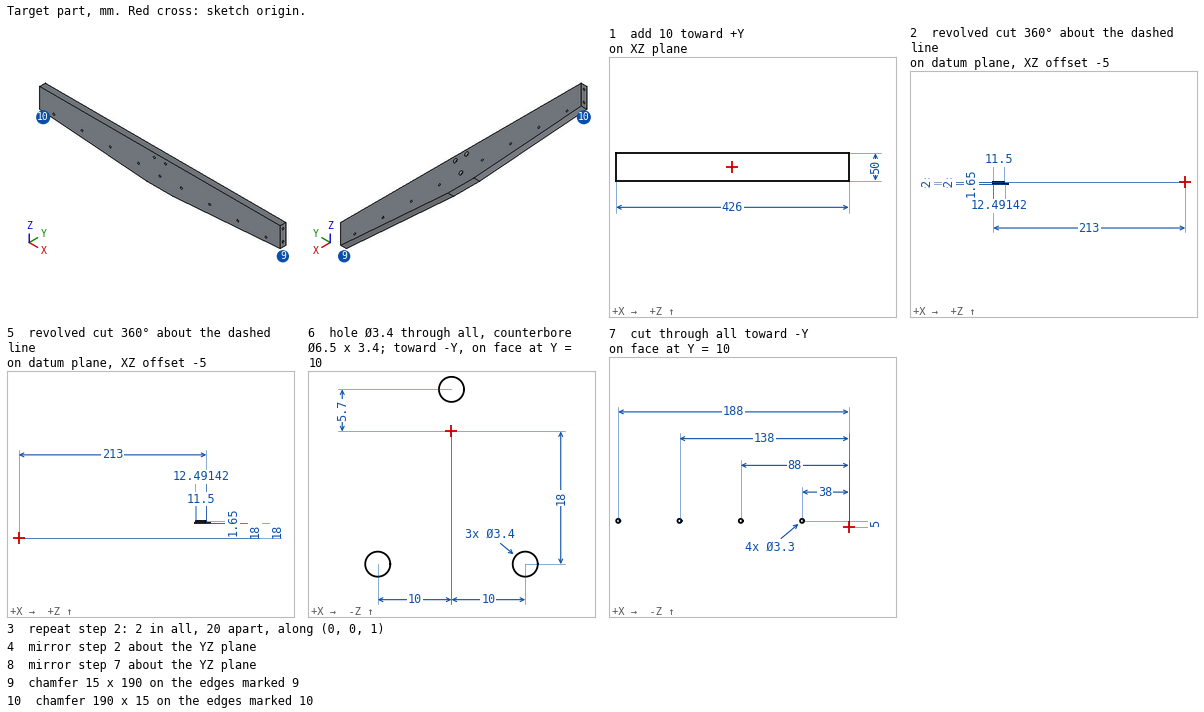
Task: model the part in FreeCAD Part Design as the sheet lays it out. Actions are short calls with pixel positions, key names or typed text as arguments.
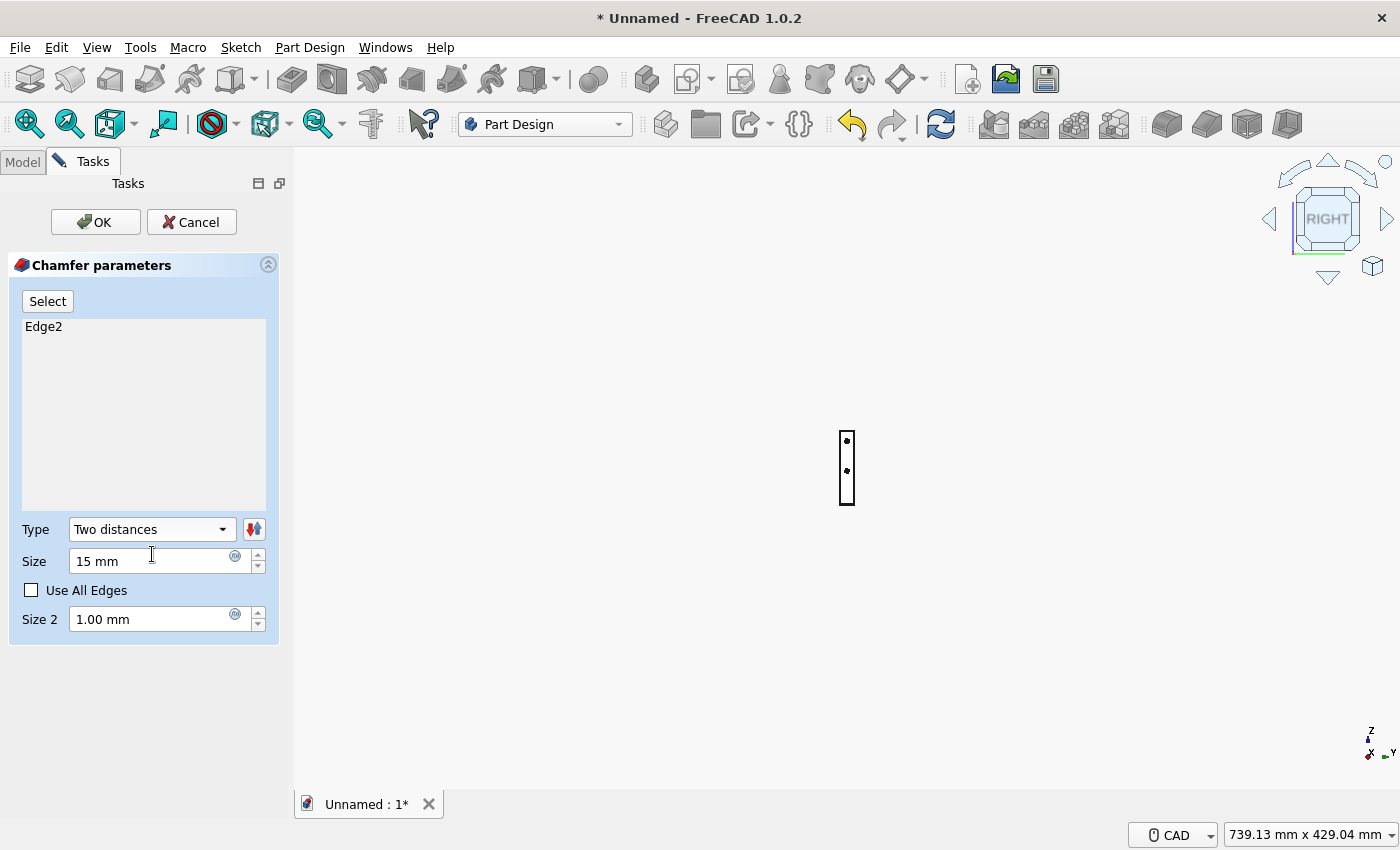
triple_click(160, 619)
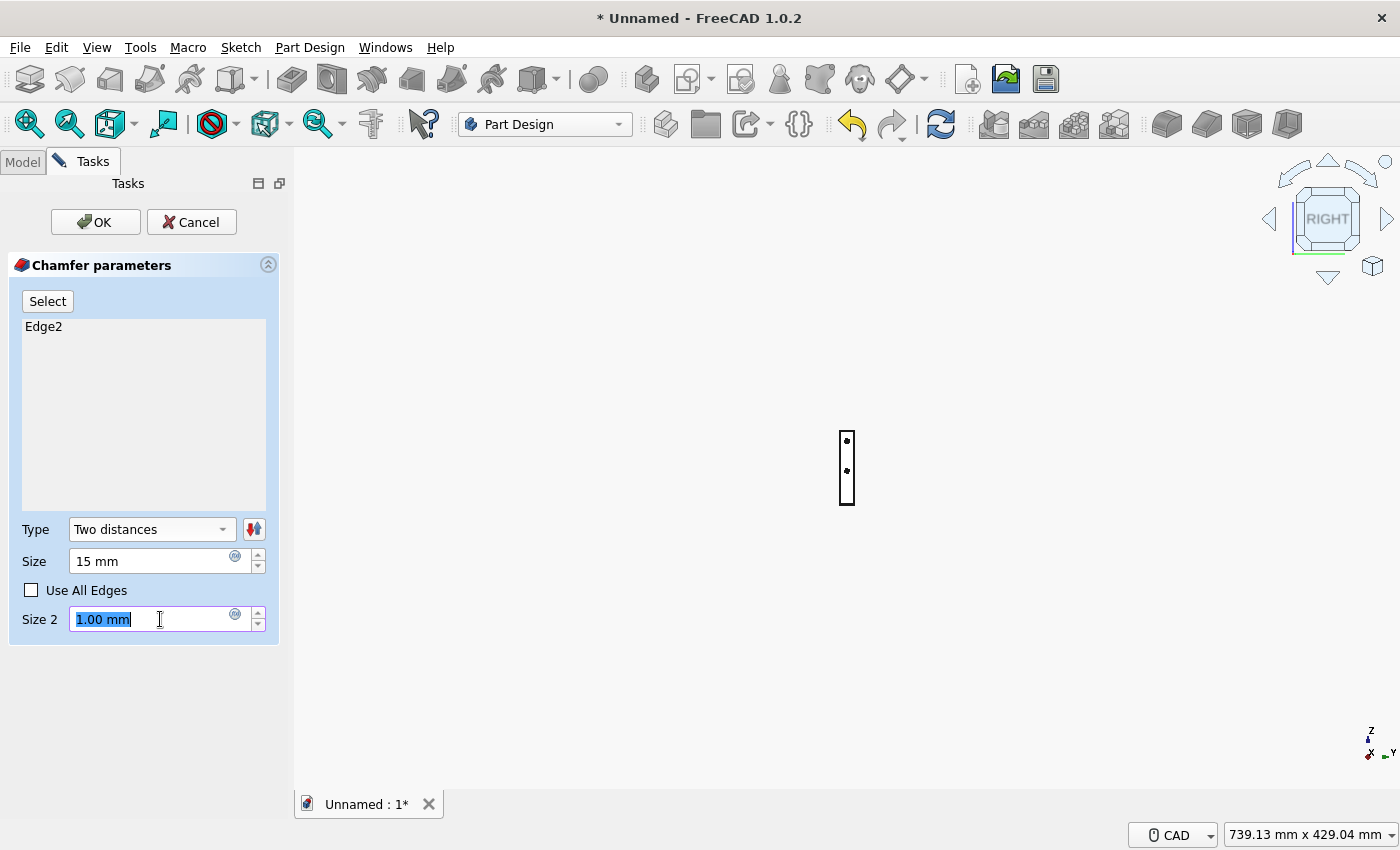
text(190)
key(Tab)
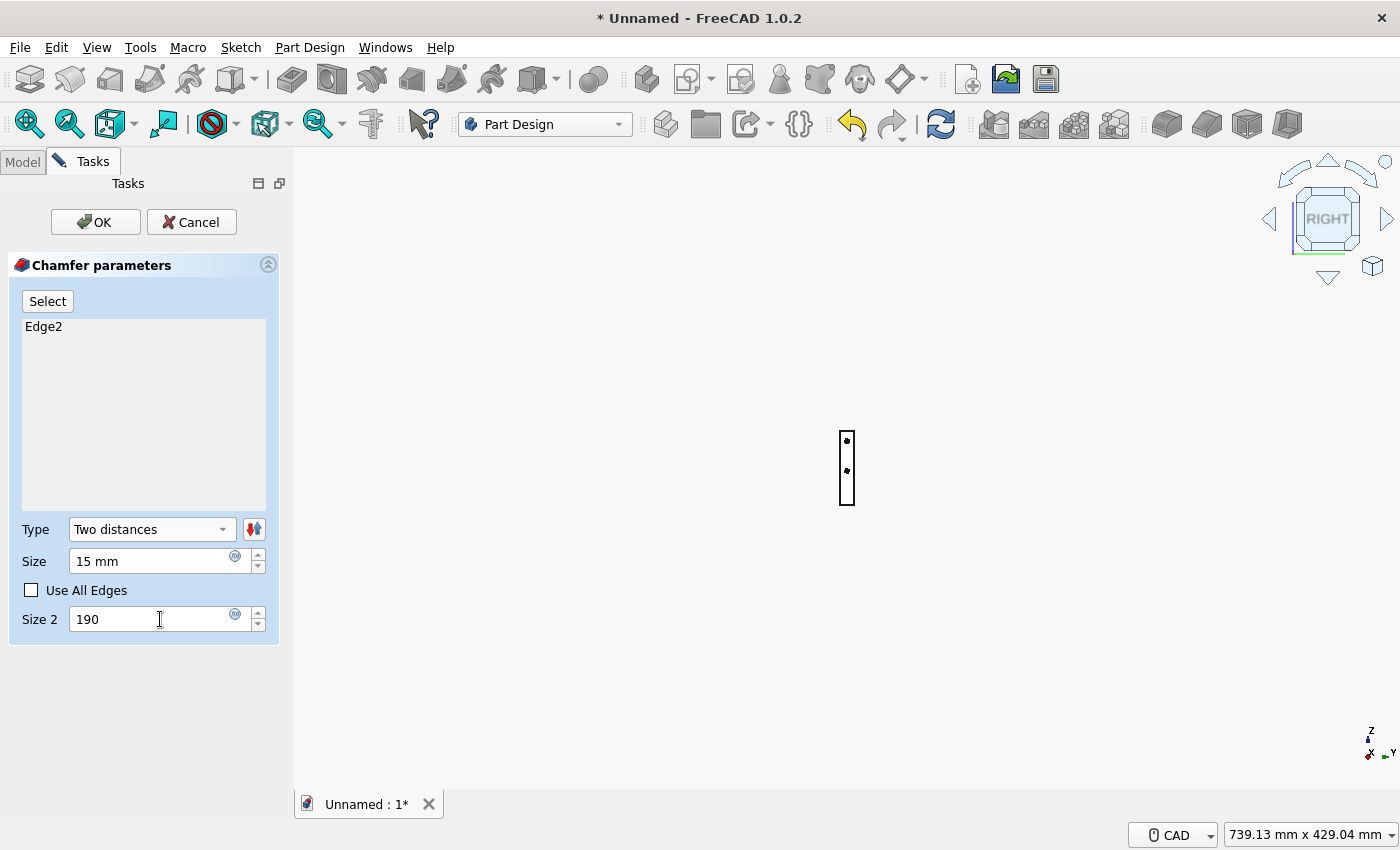
click(254, 530)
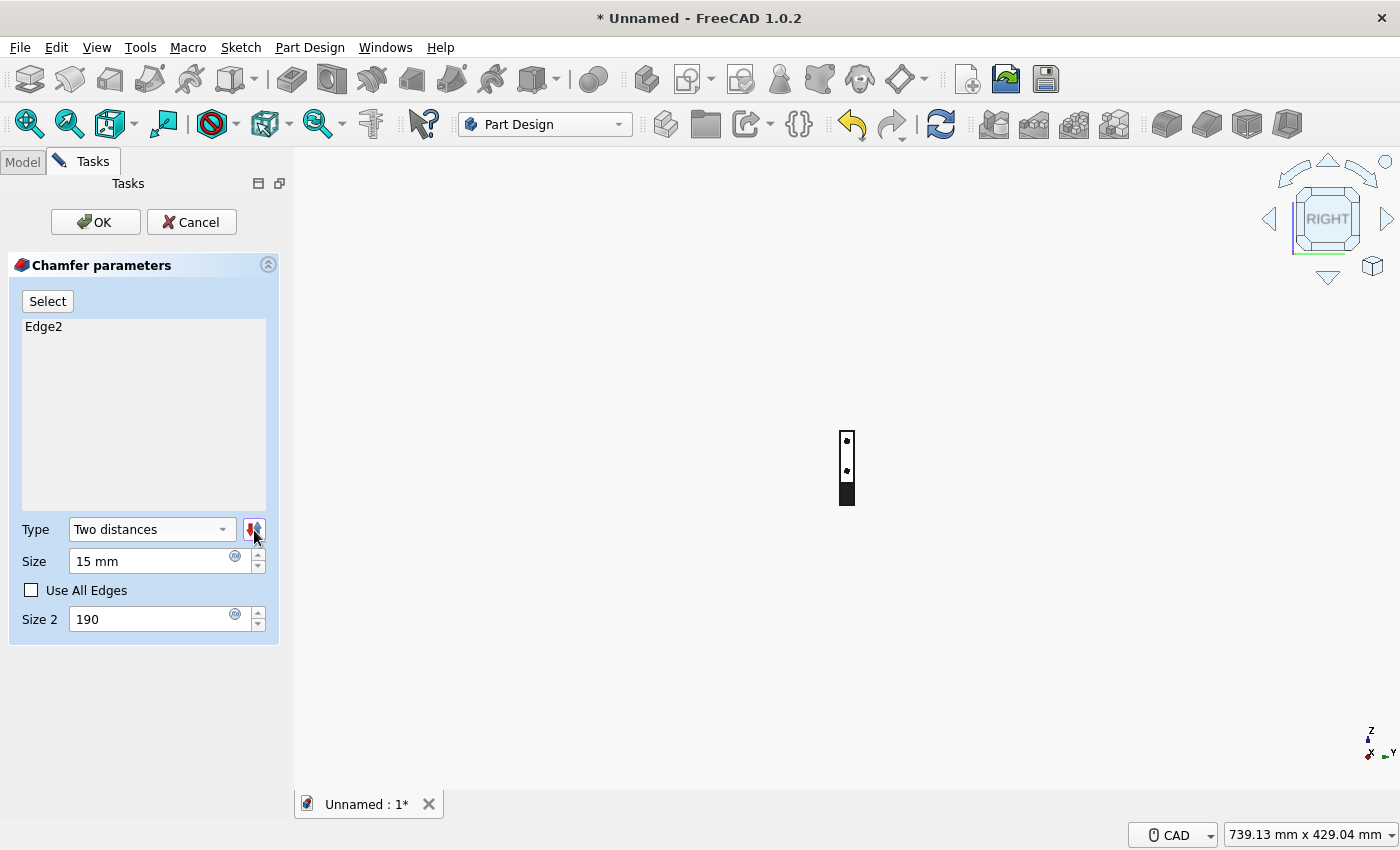
click(96, 222)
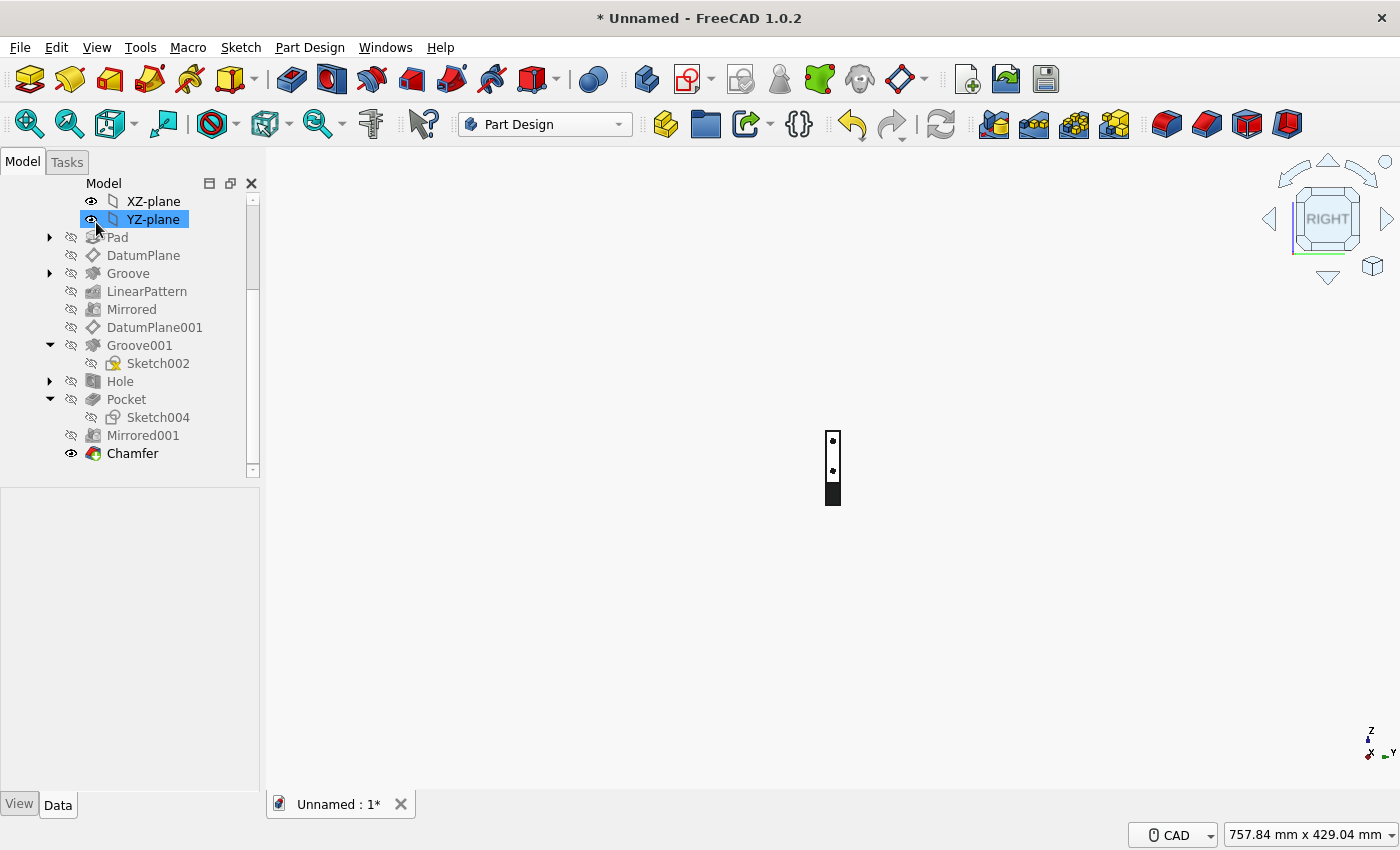
click(30, 124)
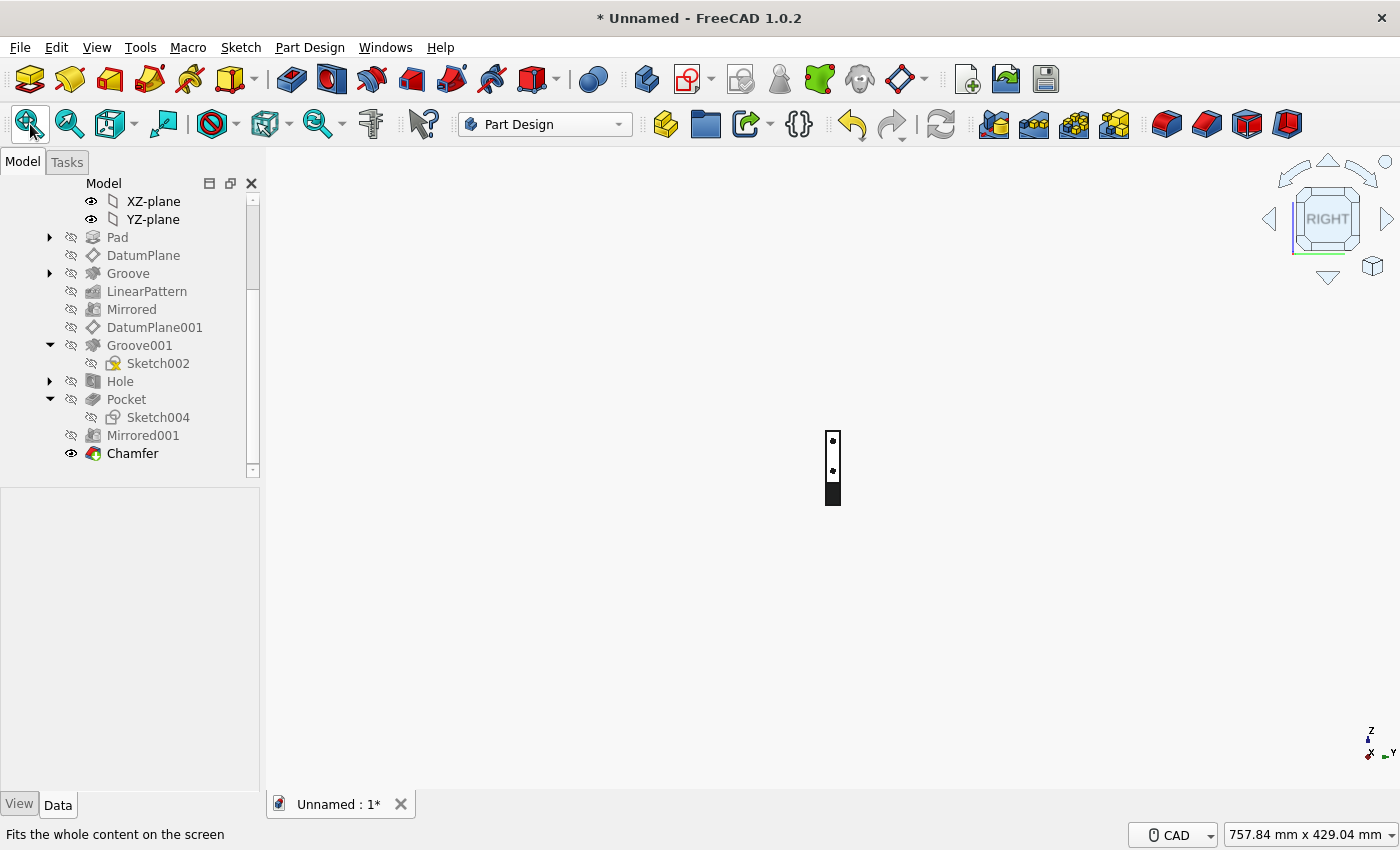
scroll(833, 504, up, 5)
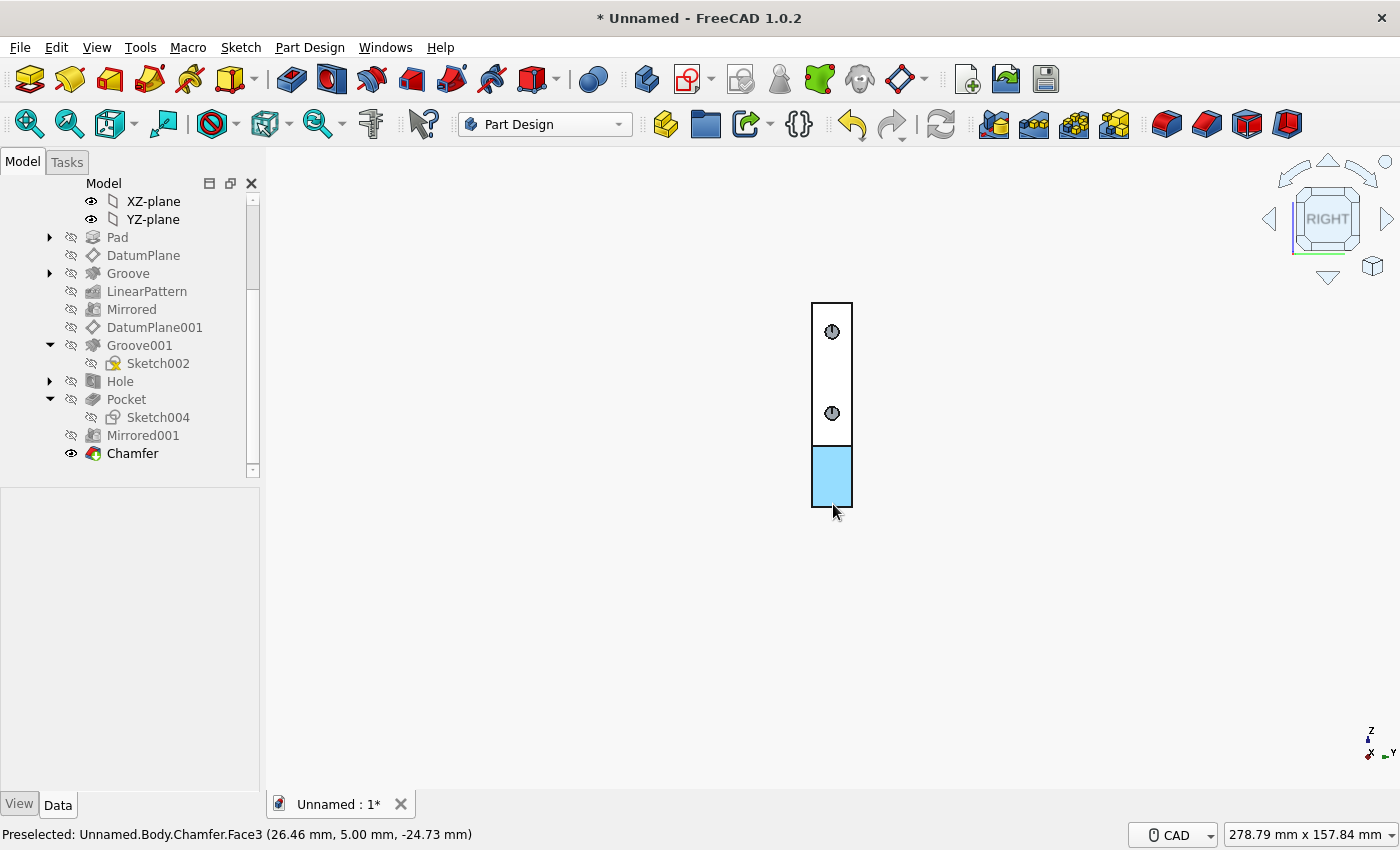
click(30, 124)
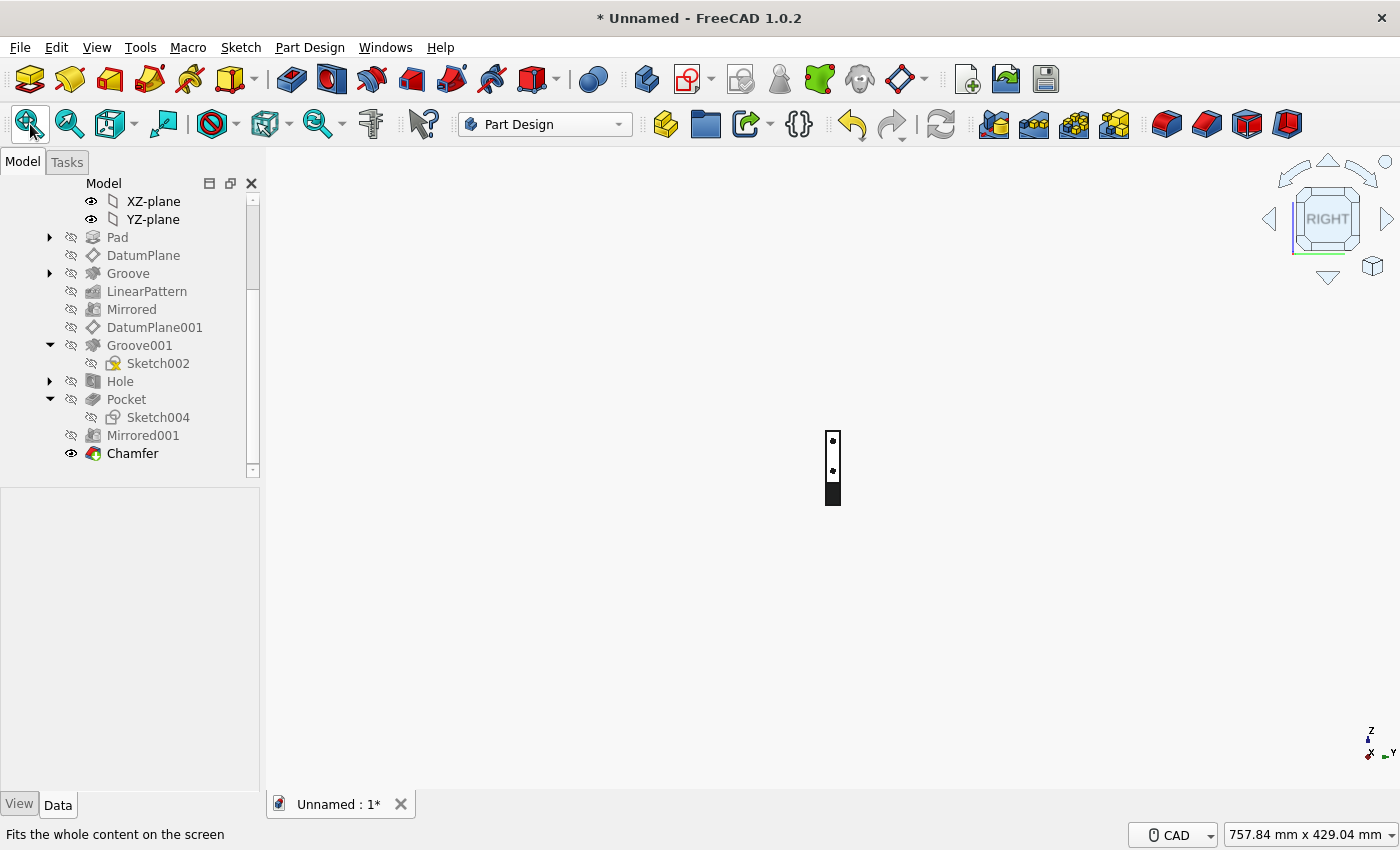
key(0)